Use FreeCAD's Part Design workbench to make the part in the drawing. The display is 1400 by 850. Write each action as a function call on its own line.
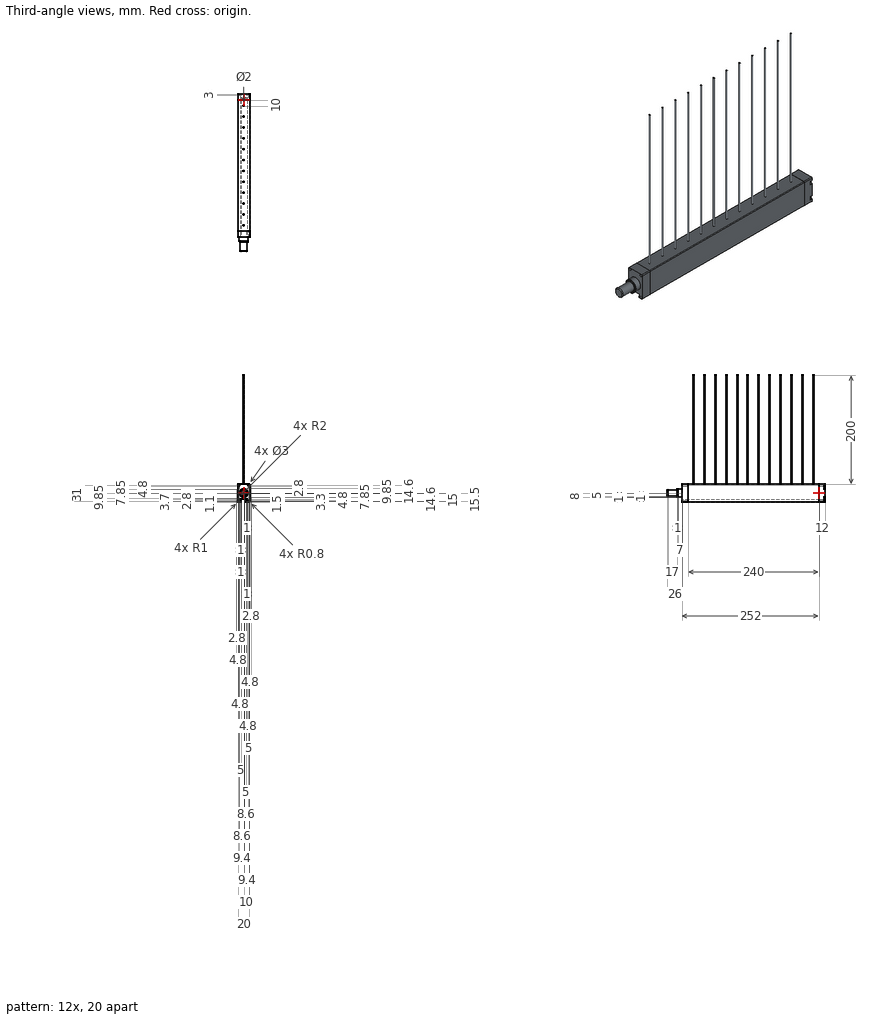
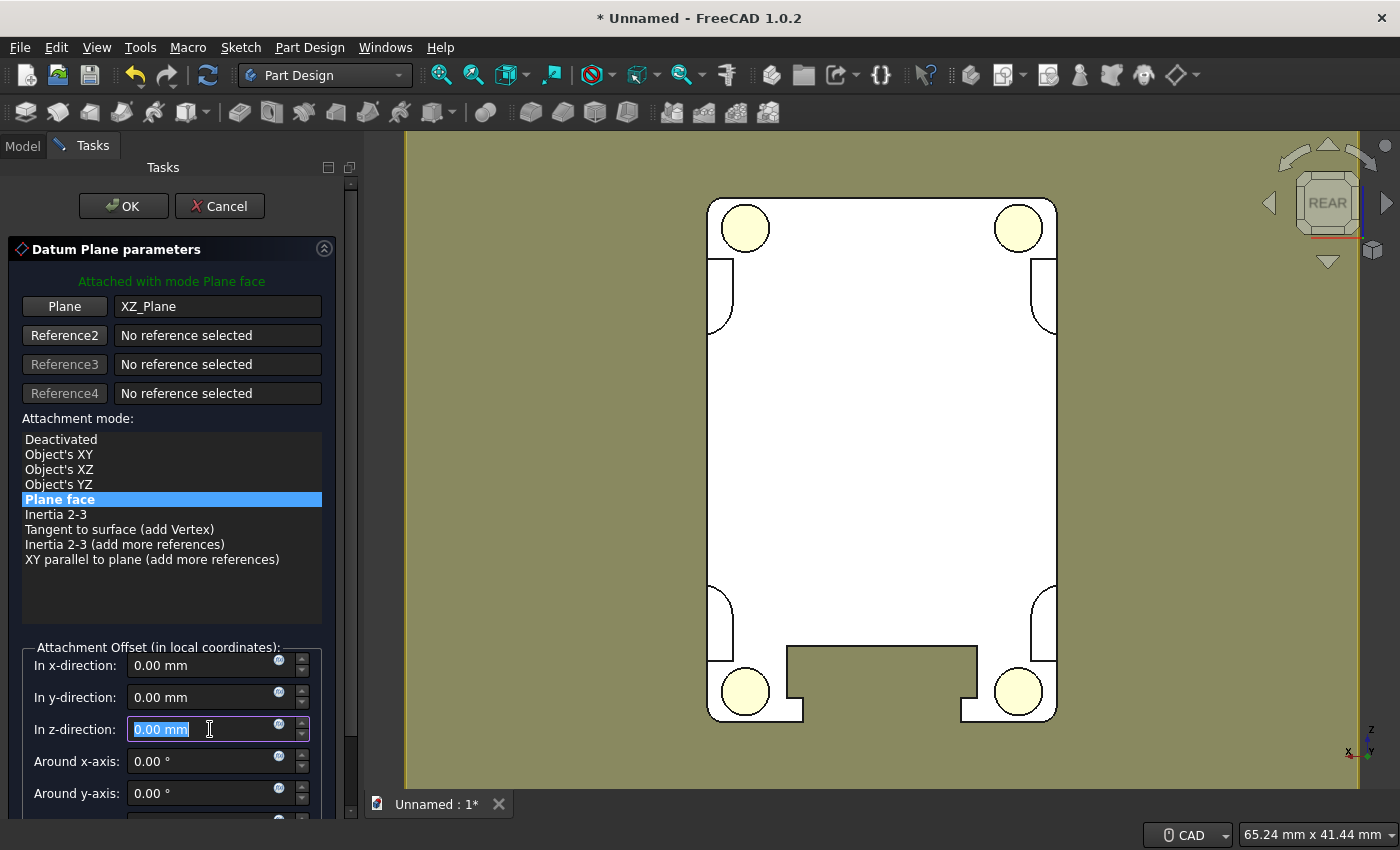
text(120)
key(Tab)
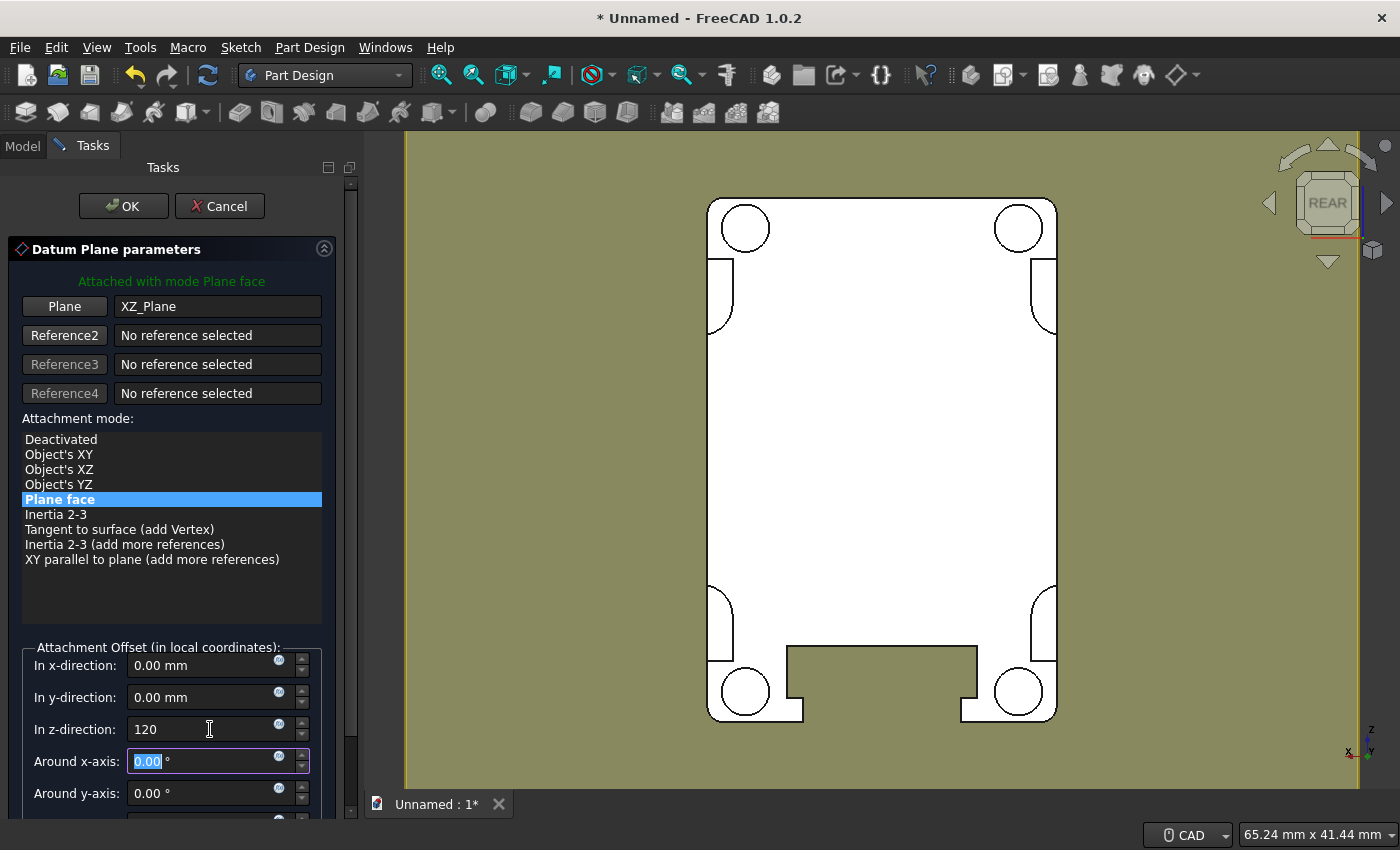
click(124, 206)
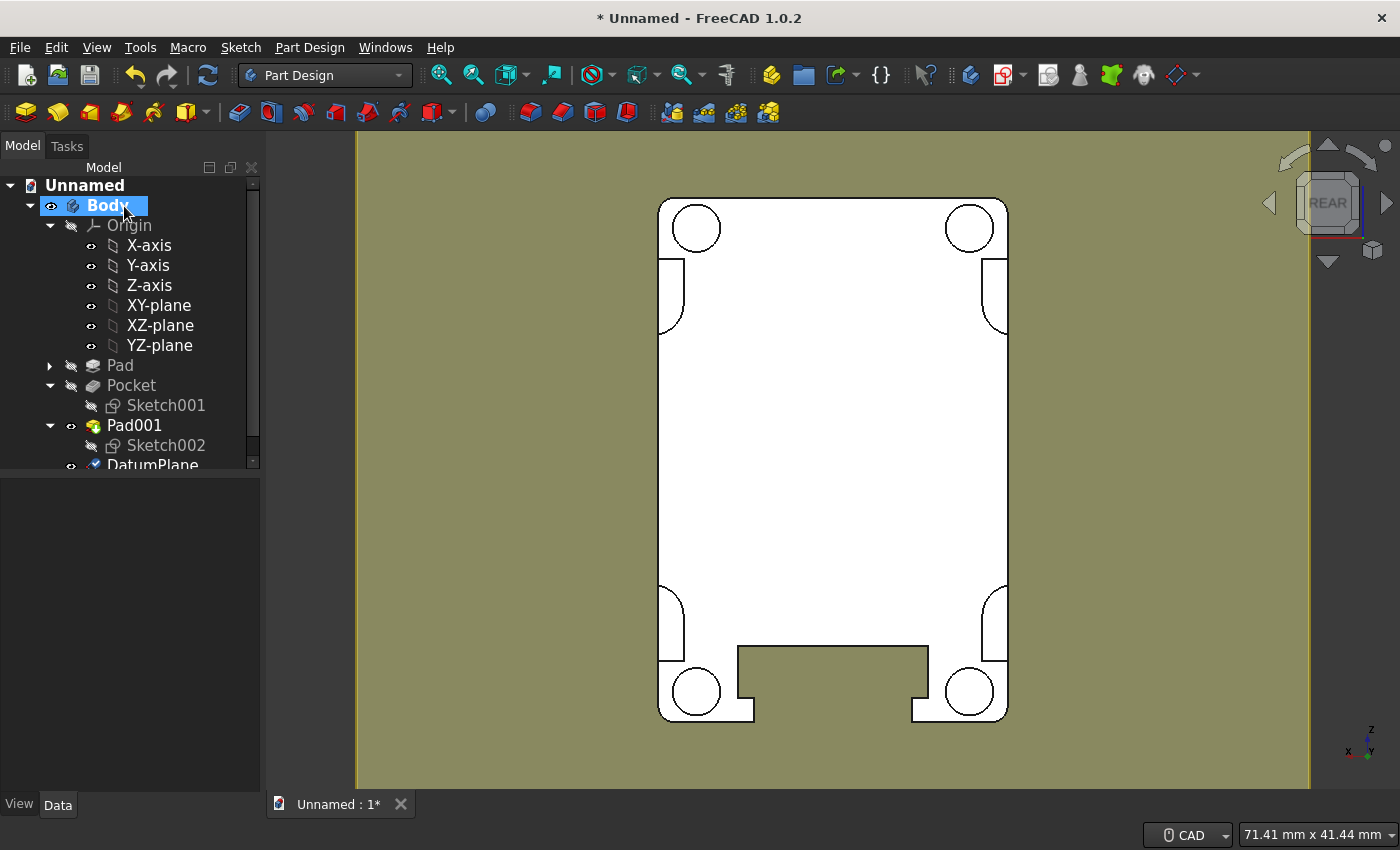
click(116, 366)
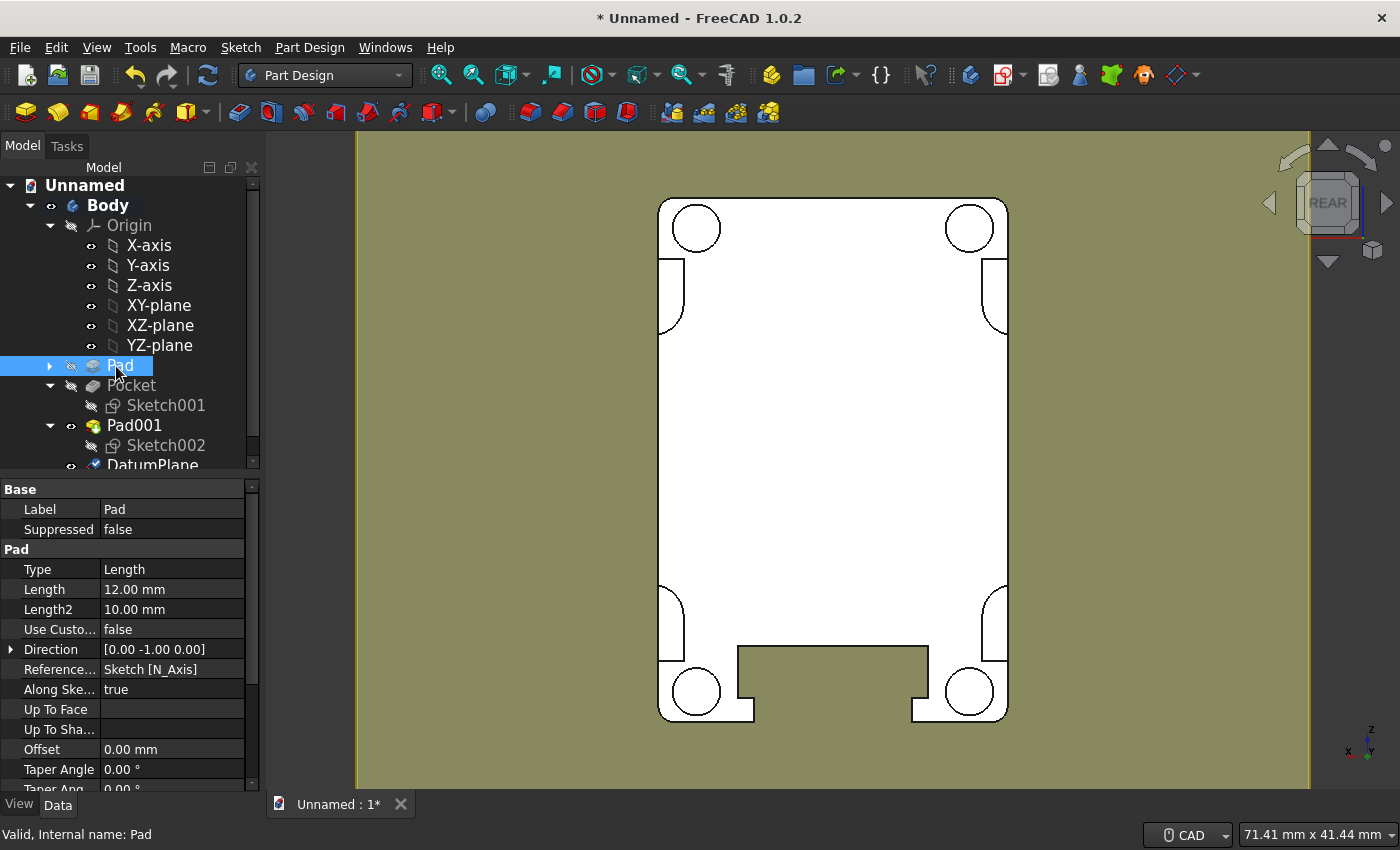
click(672, 112)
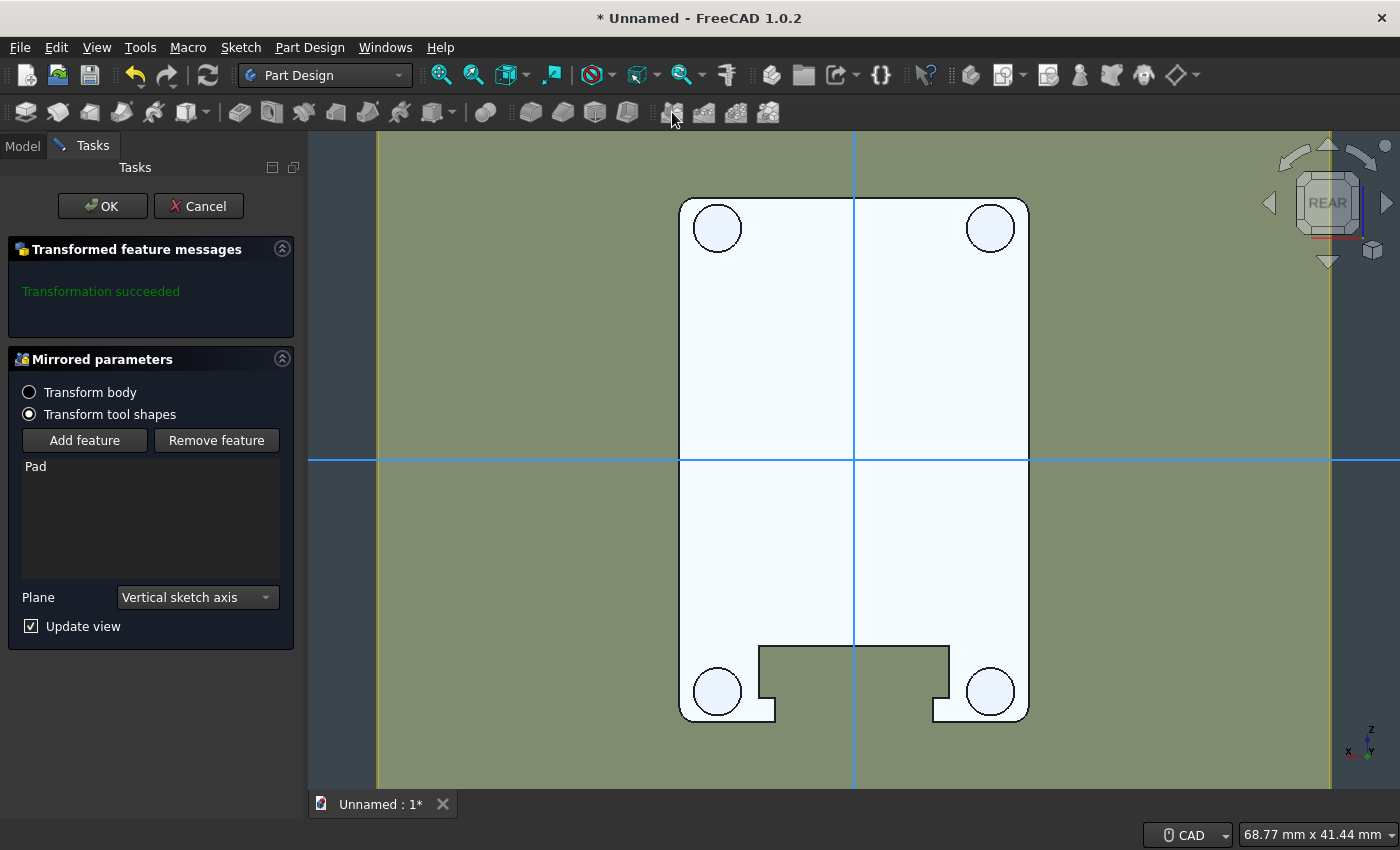
click(198, 598)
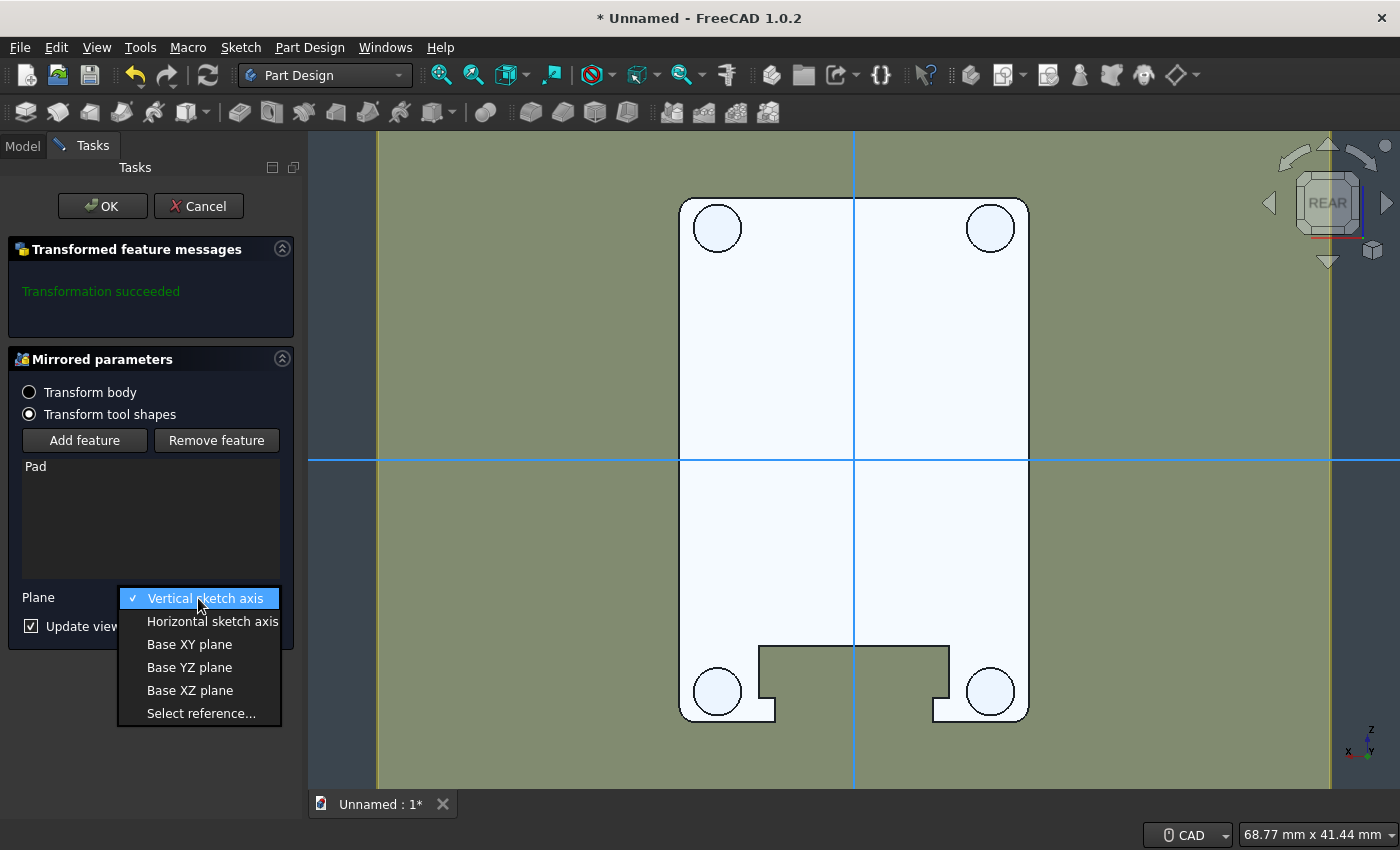
click(198, 714)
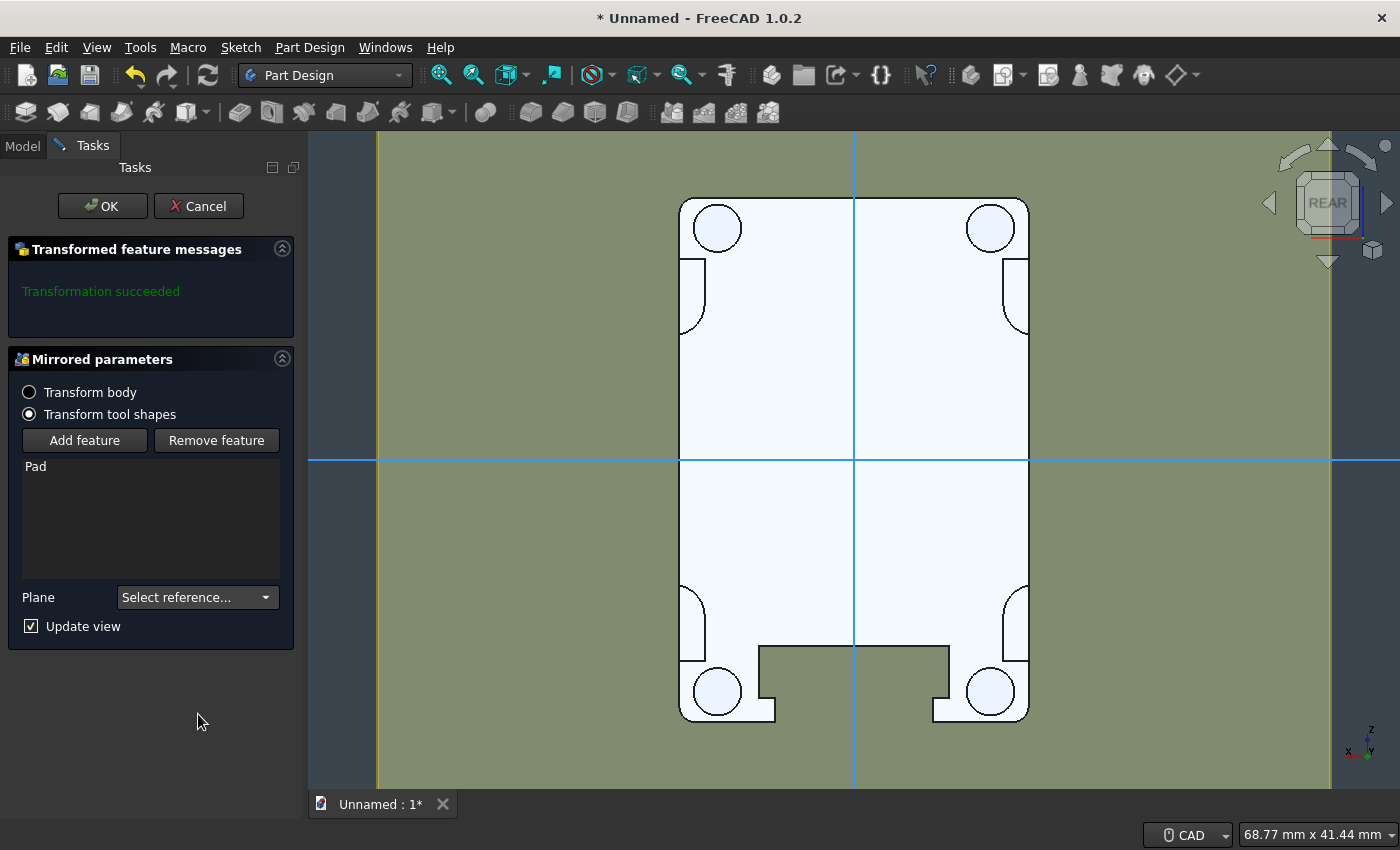
click(23, 145)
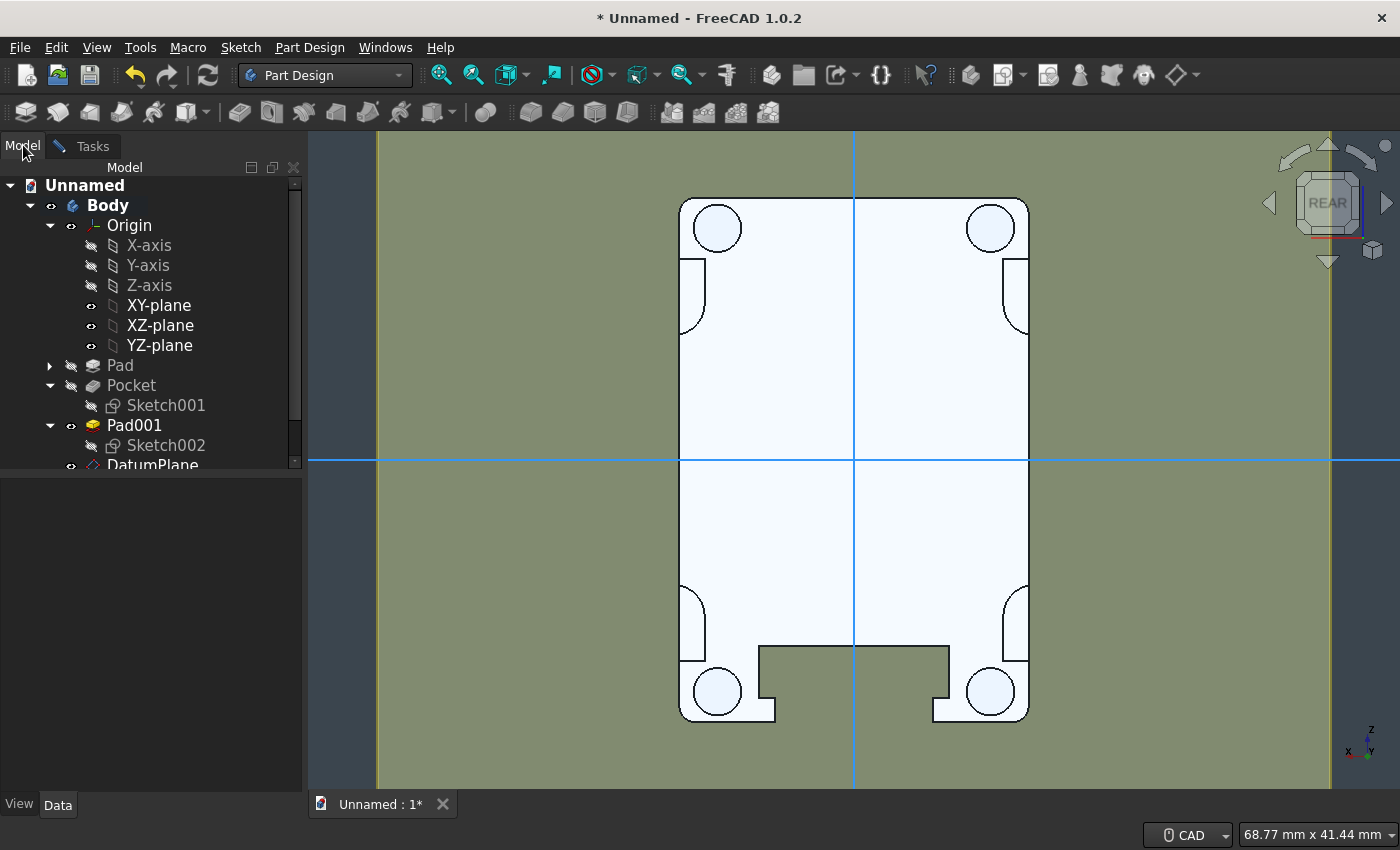
click(116, 466)